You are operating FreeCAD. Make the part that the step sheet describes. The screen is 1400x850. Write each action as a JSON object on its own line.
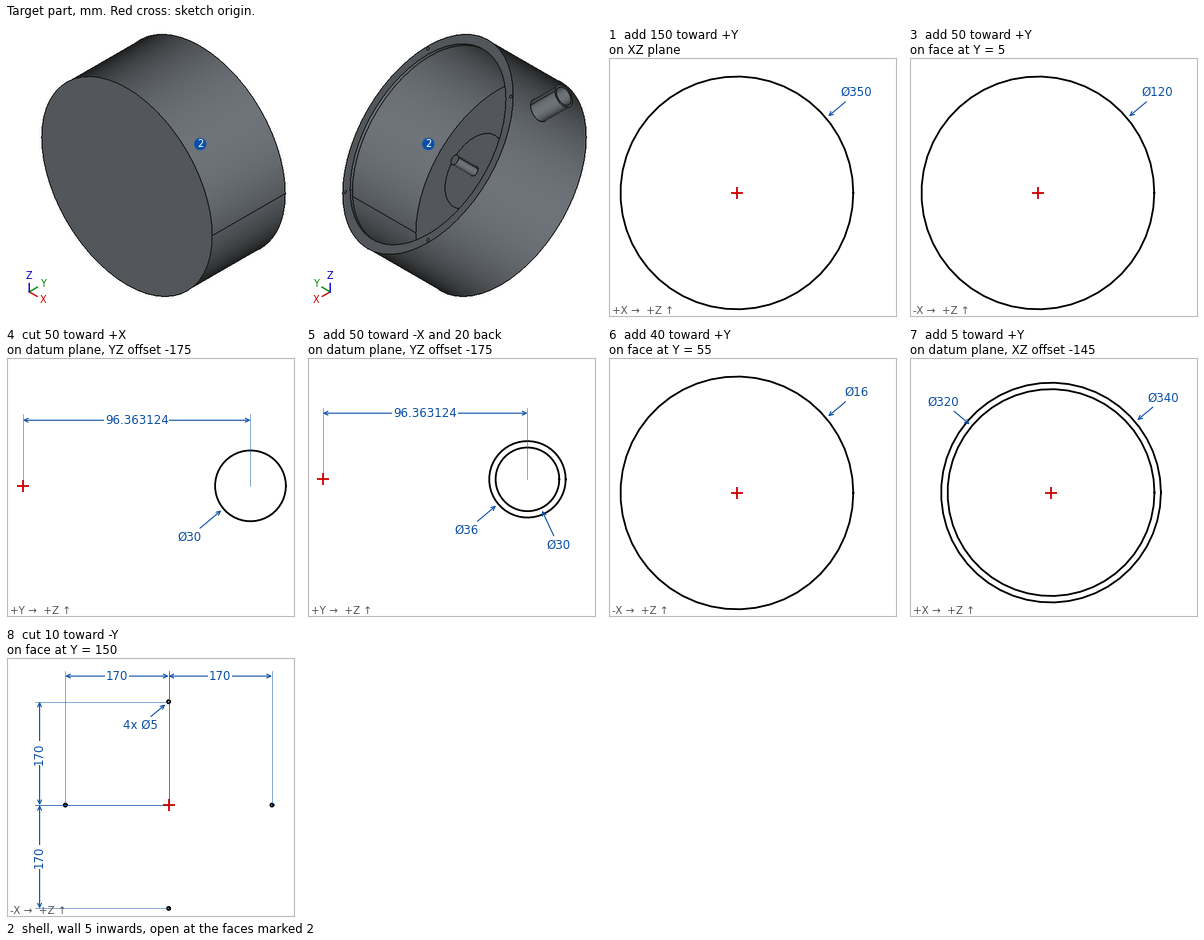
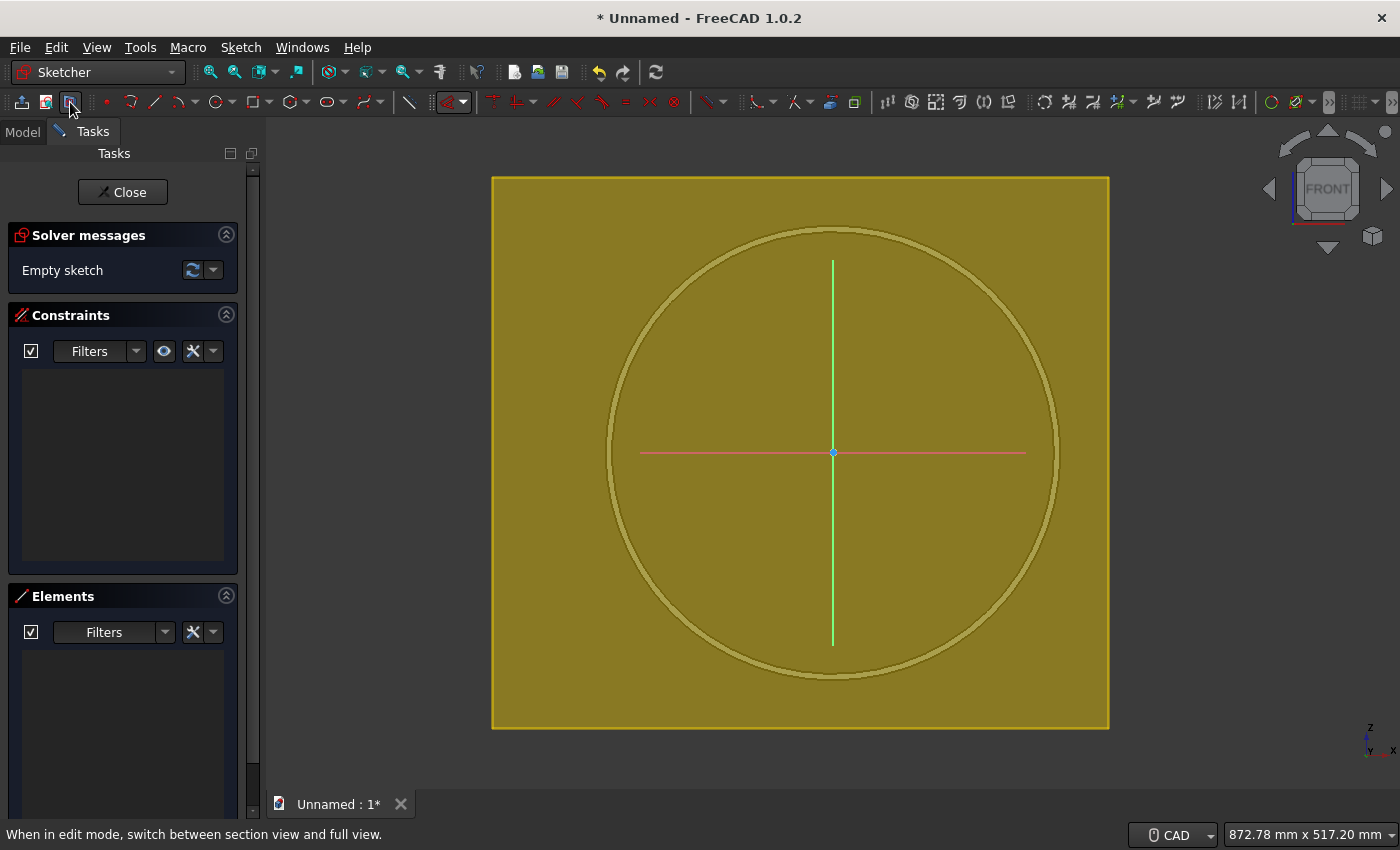
{"action": "left_click", "coordinate": [216, 102]}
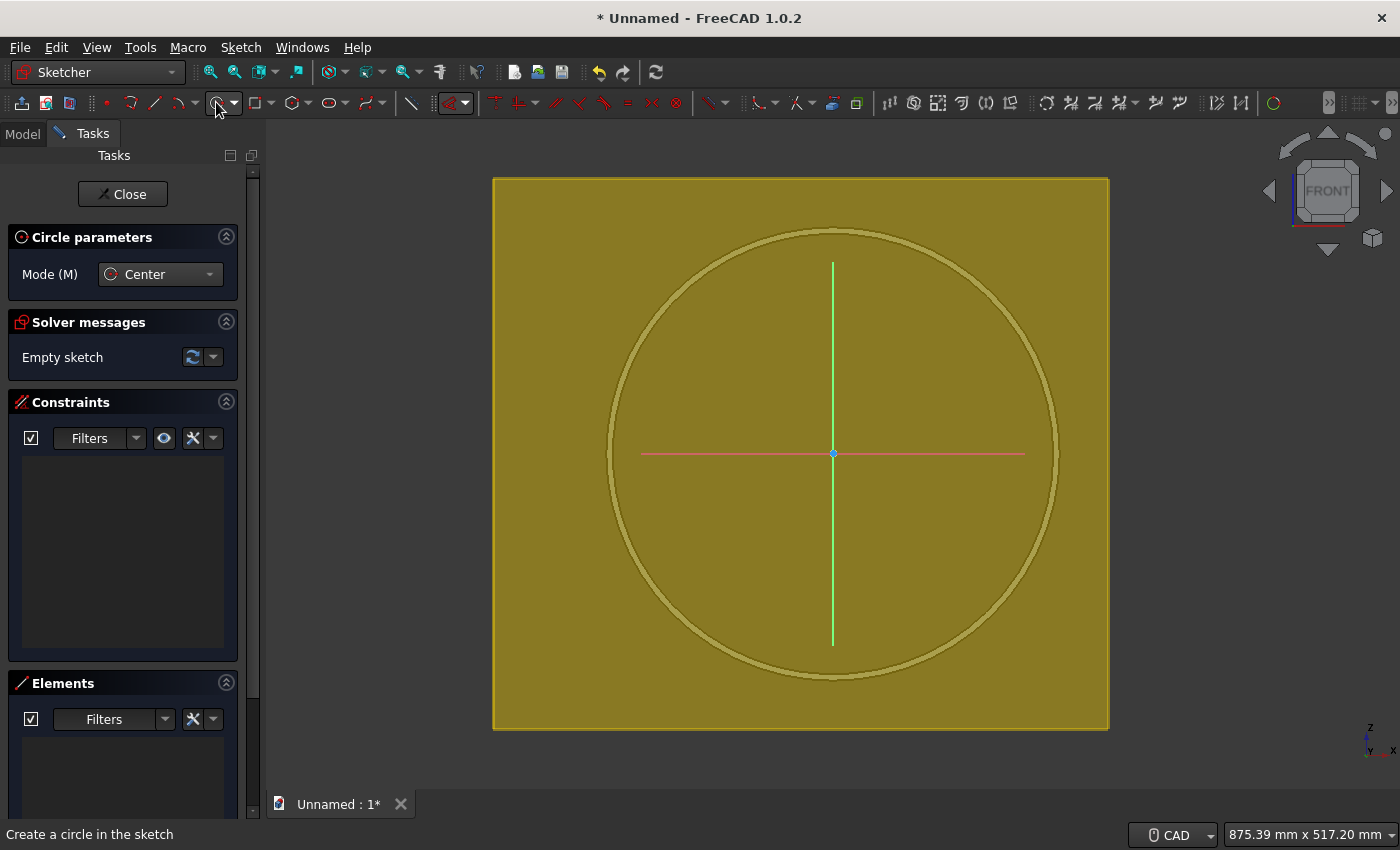
{"action": "left_click", "coordinate": [833, 454]}
{"action": "mouse_move", "coordinate": [989, 298]}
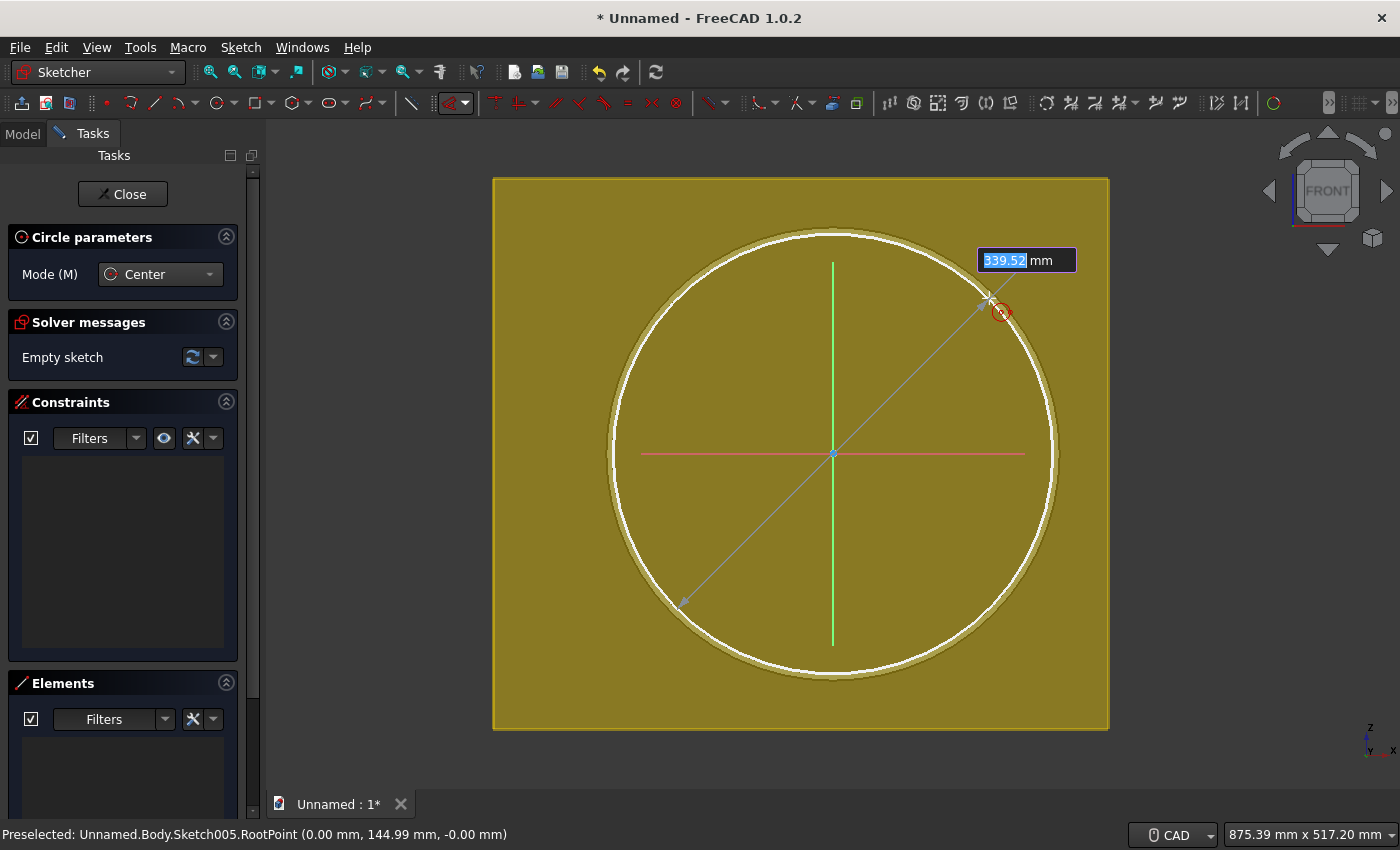
{"action": "type", "text": "340"}
{"action": "key", "text": "Return"}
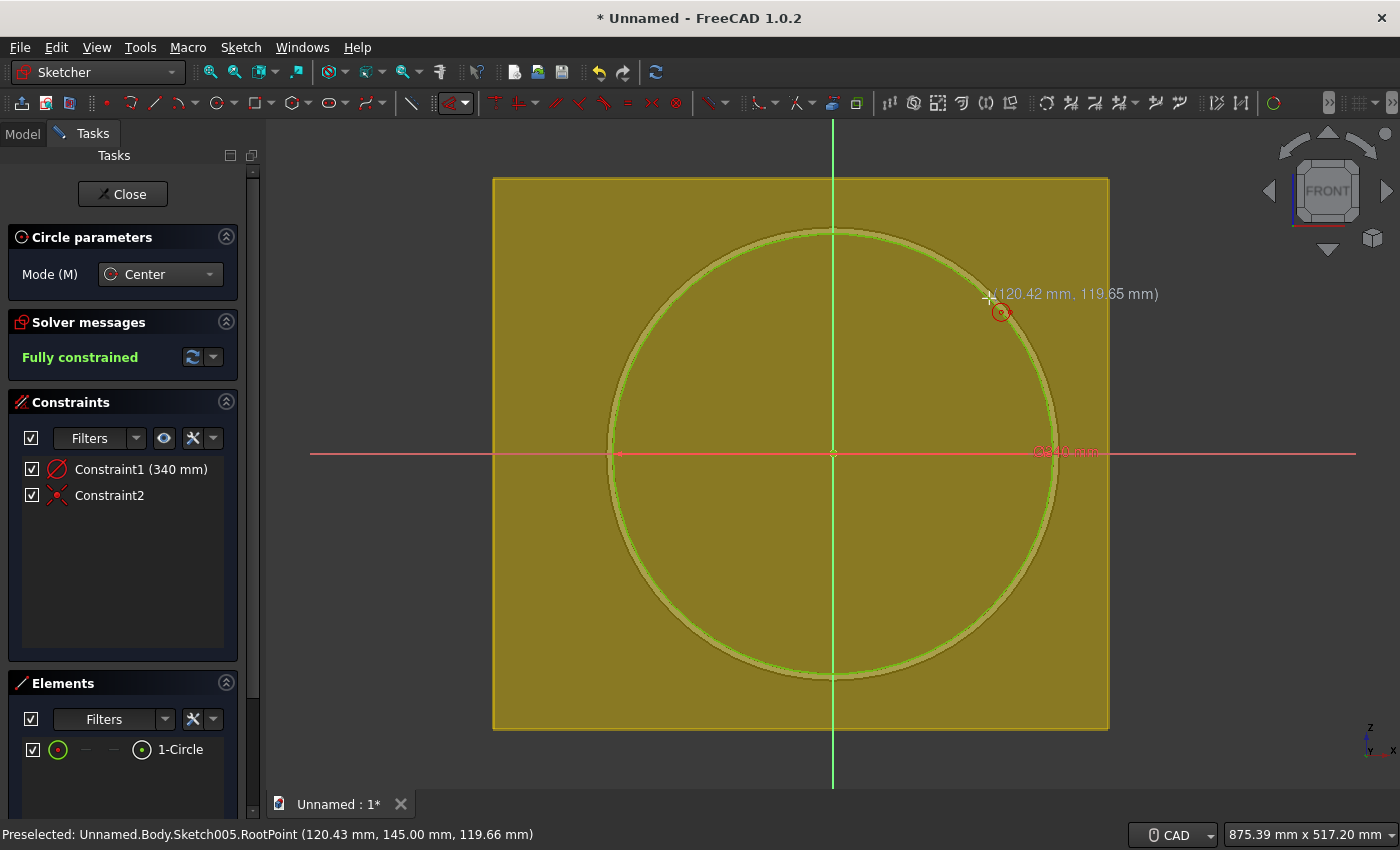
{"action": "left_click", "coordinate": [833, 454]}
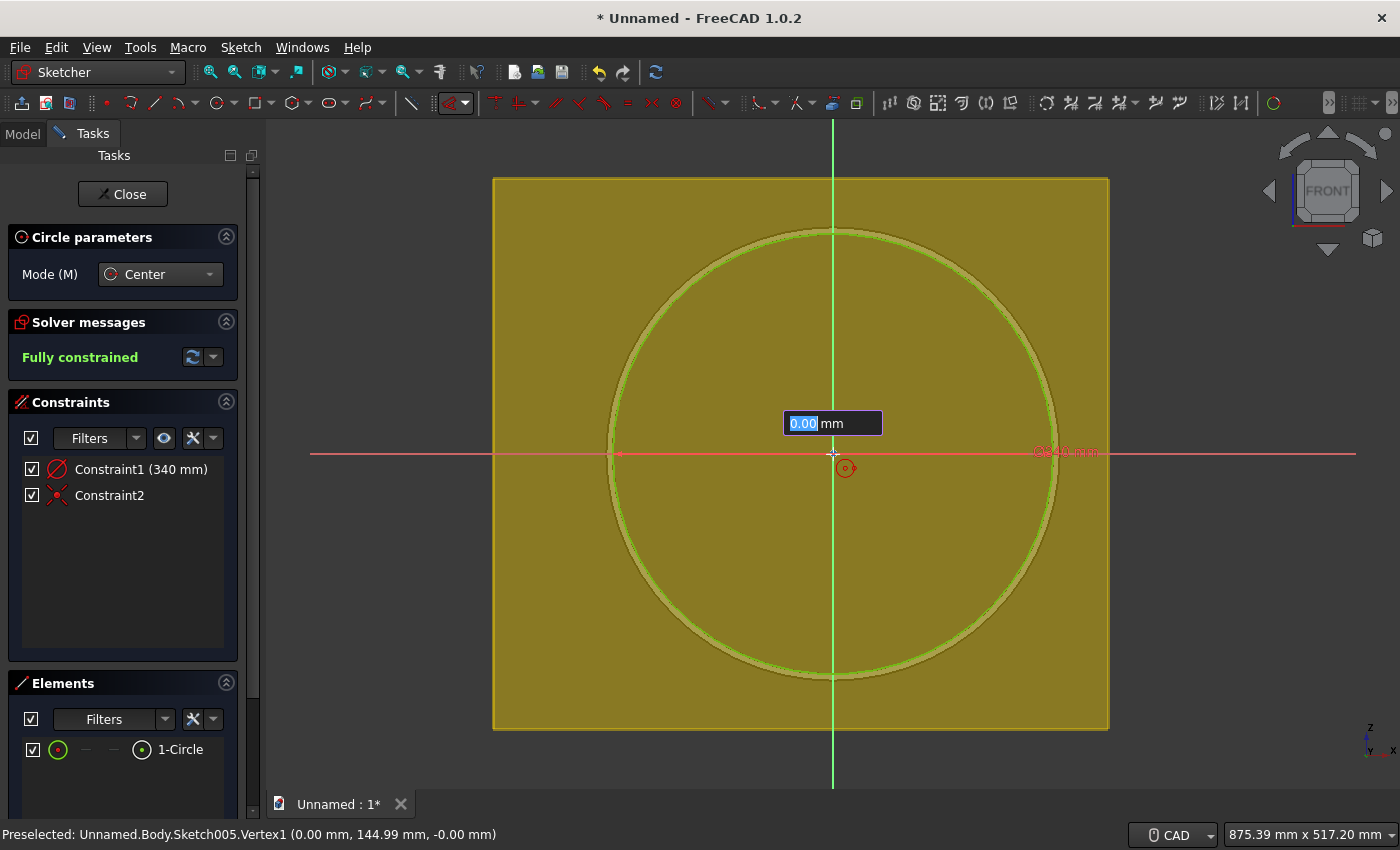
{"action": "scroll", "coordinate": [980, 307], "scroll_direction": "up", "scroll_amount": 2}
{"action": "mouse_move", "coordinate": [979, 308]}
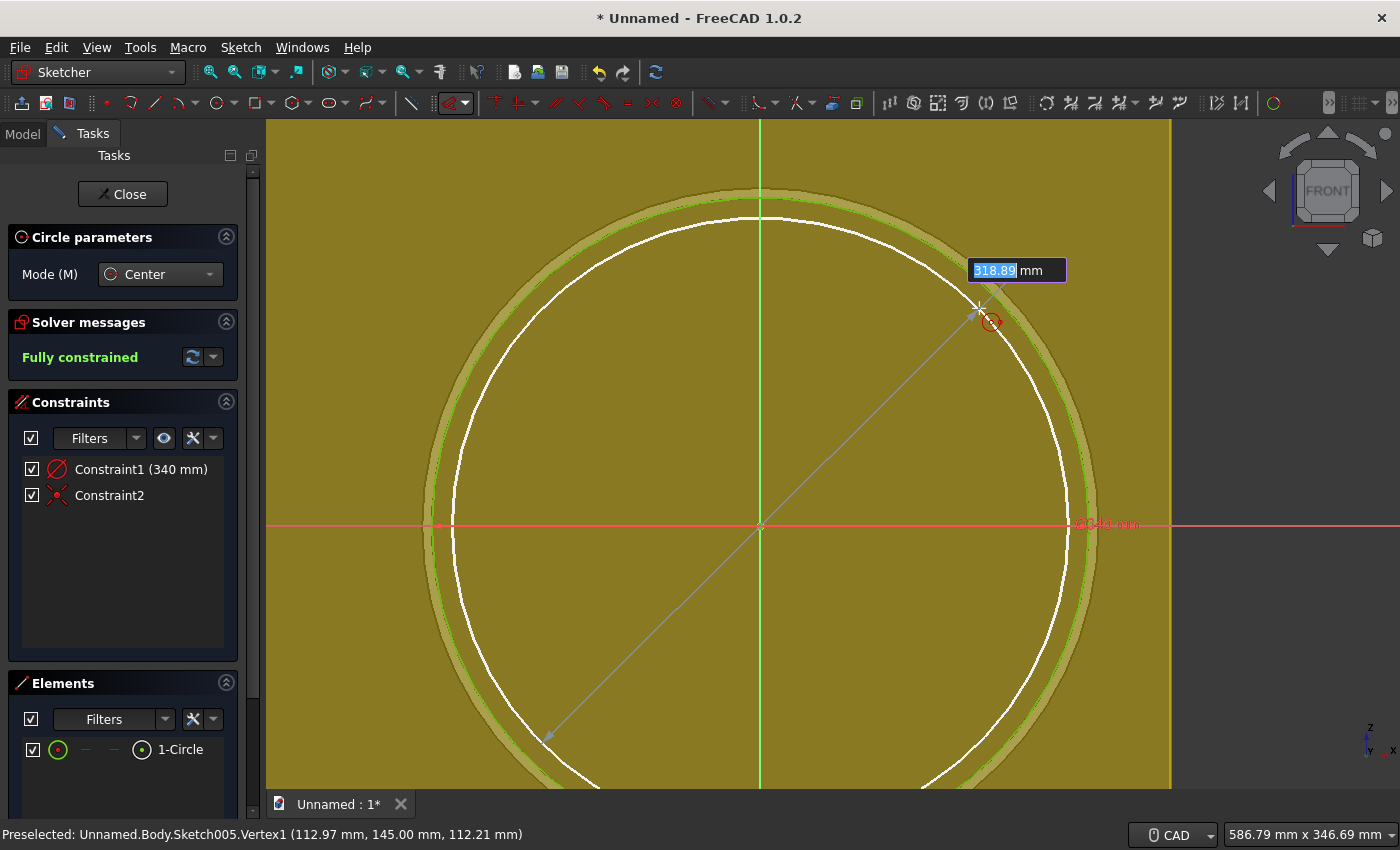
{"action": "type", "text": "320"}
{"action": "key", "text": "Return"}
{"action": "key", "text": "Escape"}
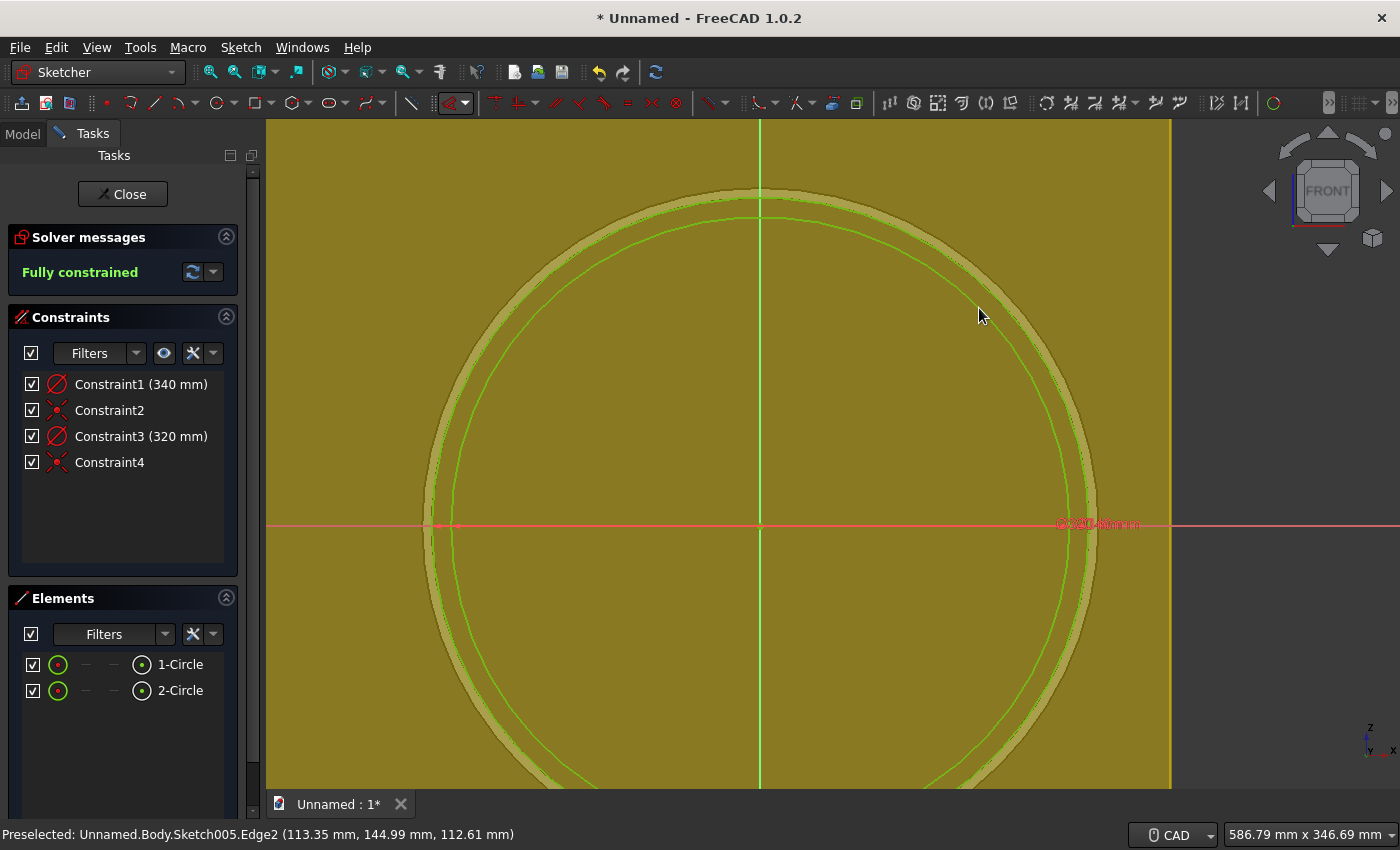
{"action": "left_click", "coordinate": [123, 194]}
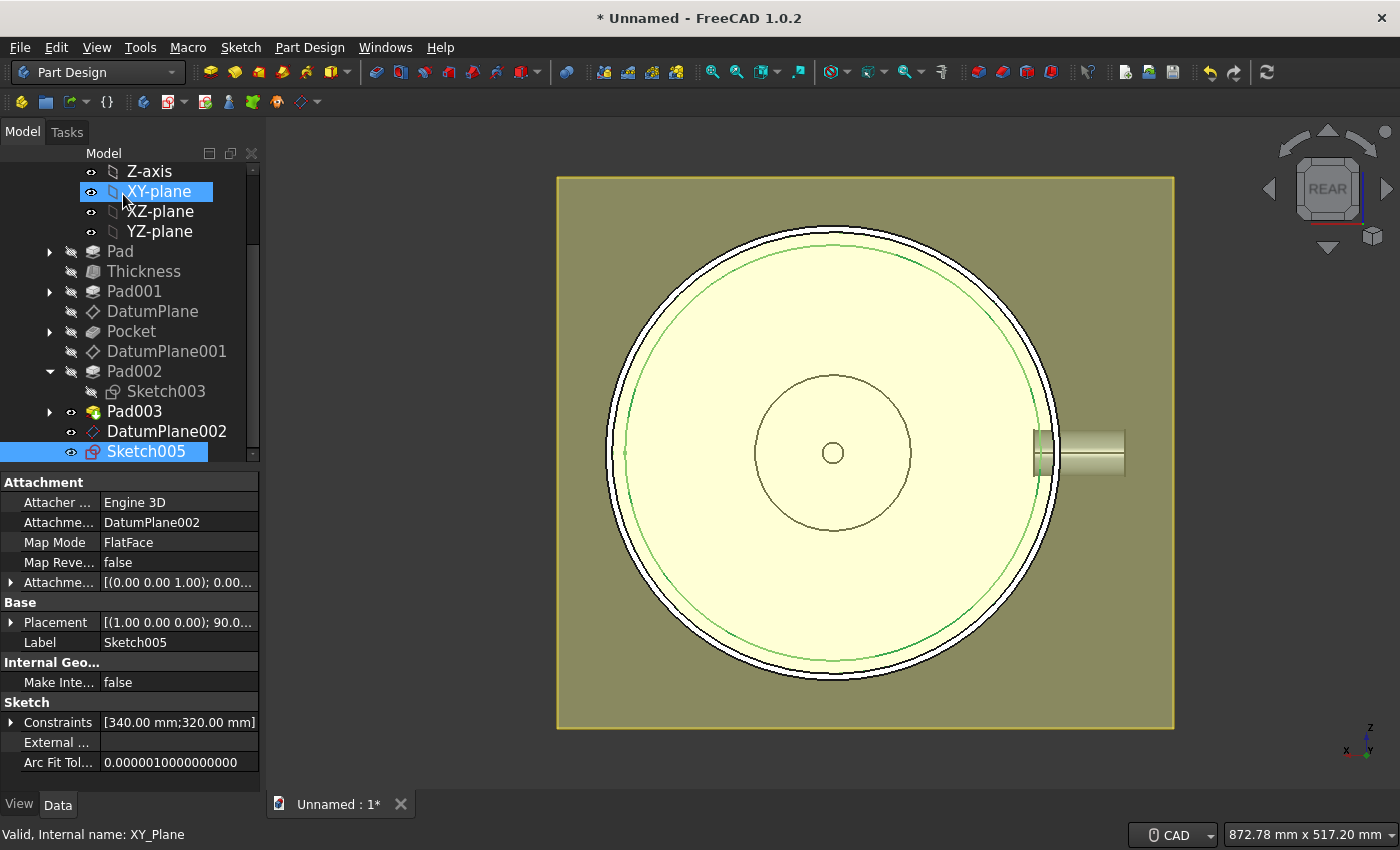
{"action": "left_click", "coordinate": [212, 72]}